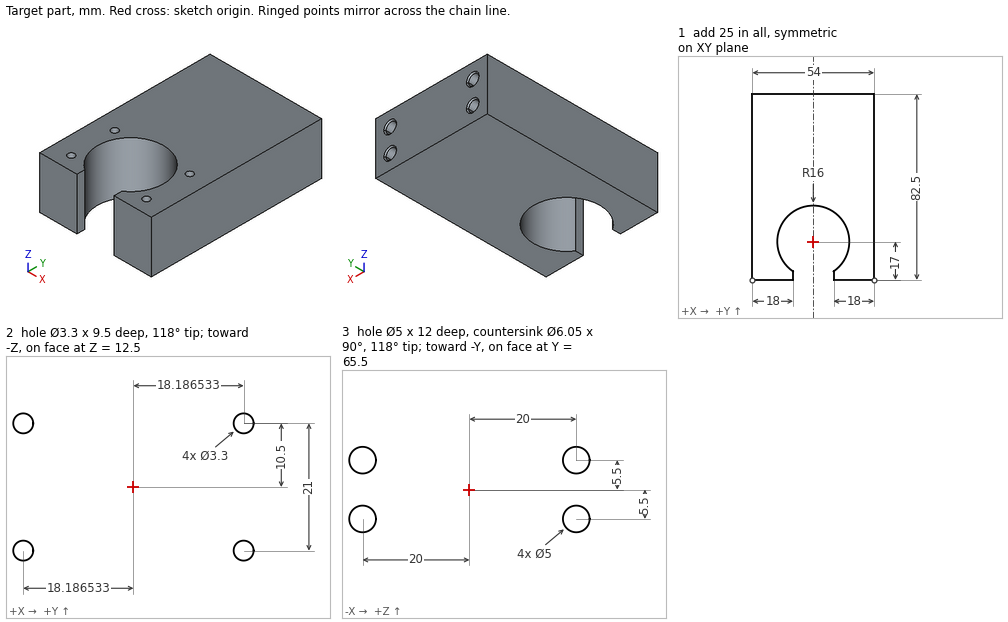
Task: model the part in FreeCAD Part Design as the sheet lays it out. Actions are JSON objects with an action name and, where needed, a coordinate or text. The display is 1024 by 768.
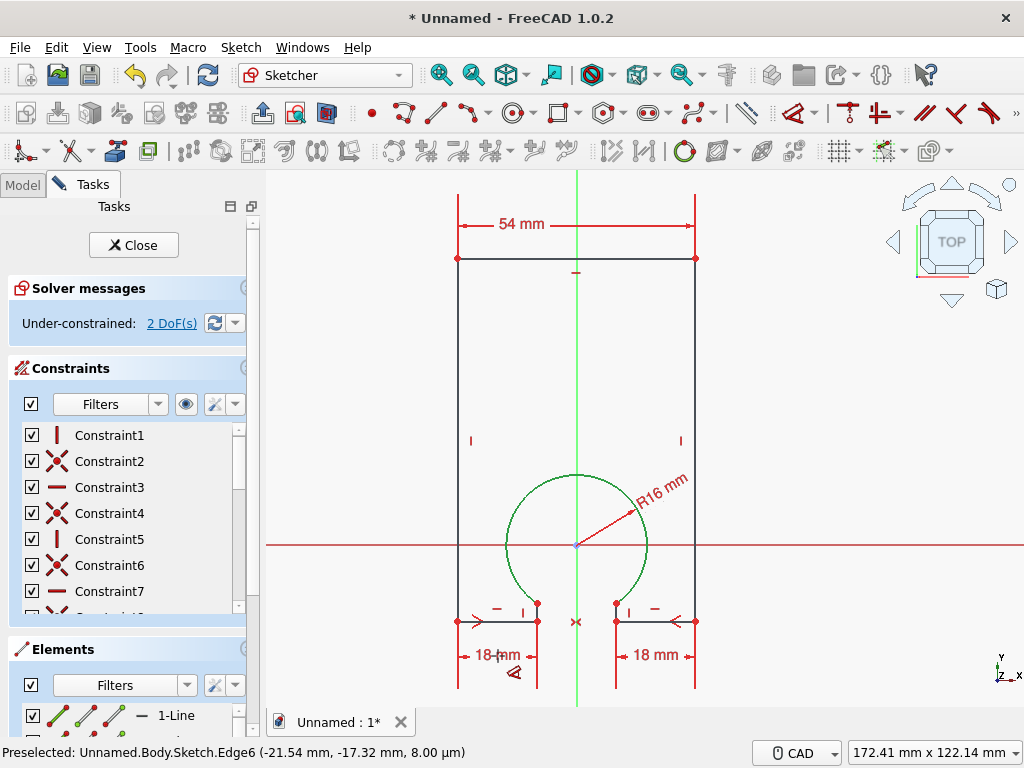
{"action": "left_click", "coordinate": [616, 622]}
{"action": "left_click", "coordinate": [650, 601]}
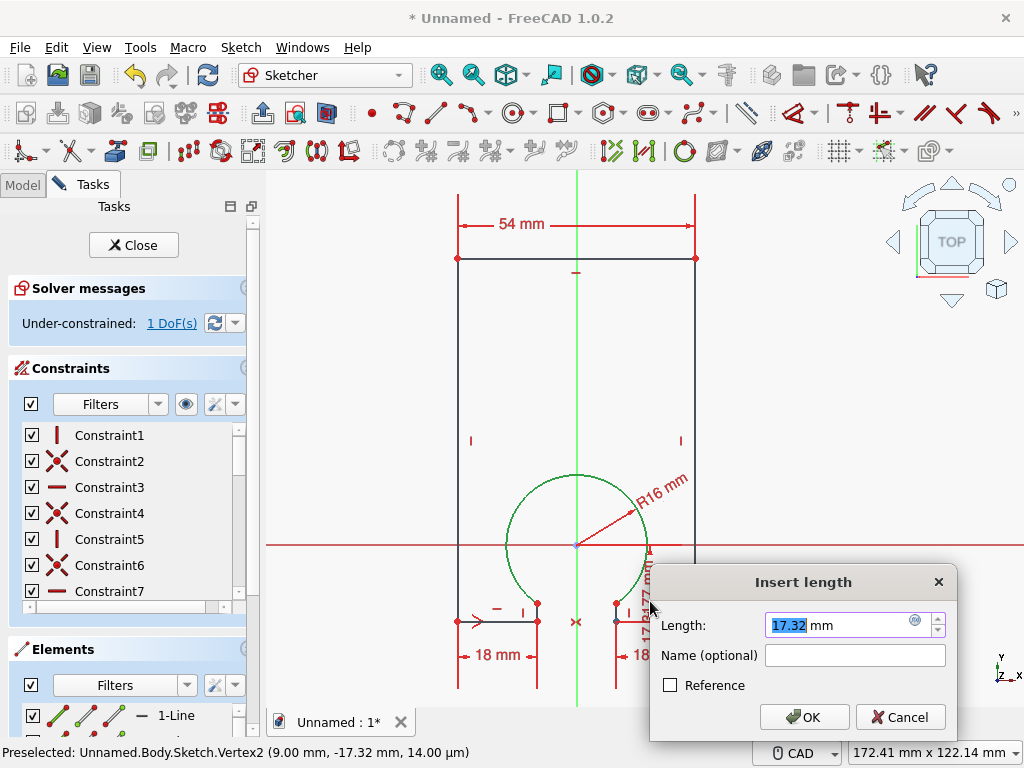
{"action": "type", "text": "17"}
{"action": "key", "text": "Return"}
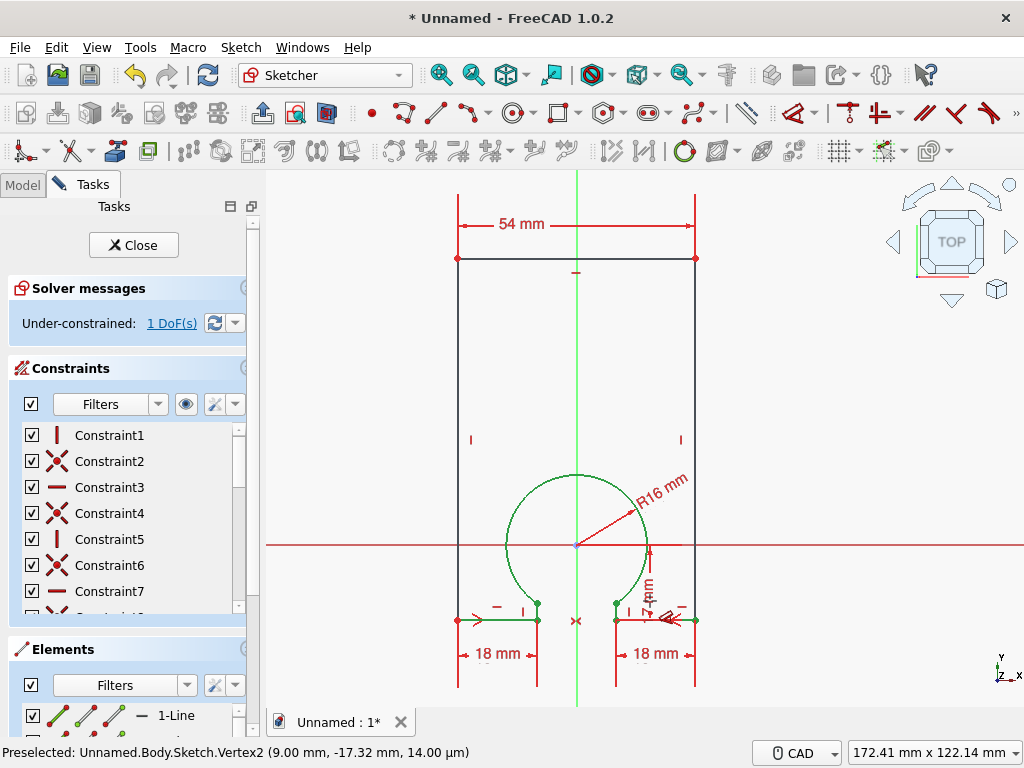
{"action": "left_click", "coordinate": [695, 512]}
{"action": "left_click", "coordinate": [729, 440]}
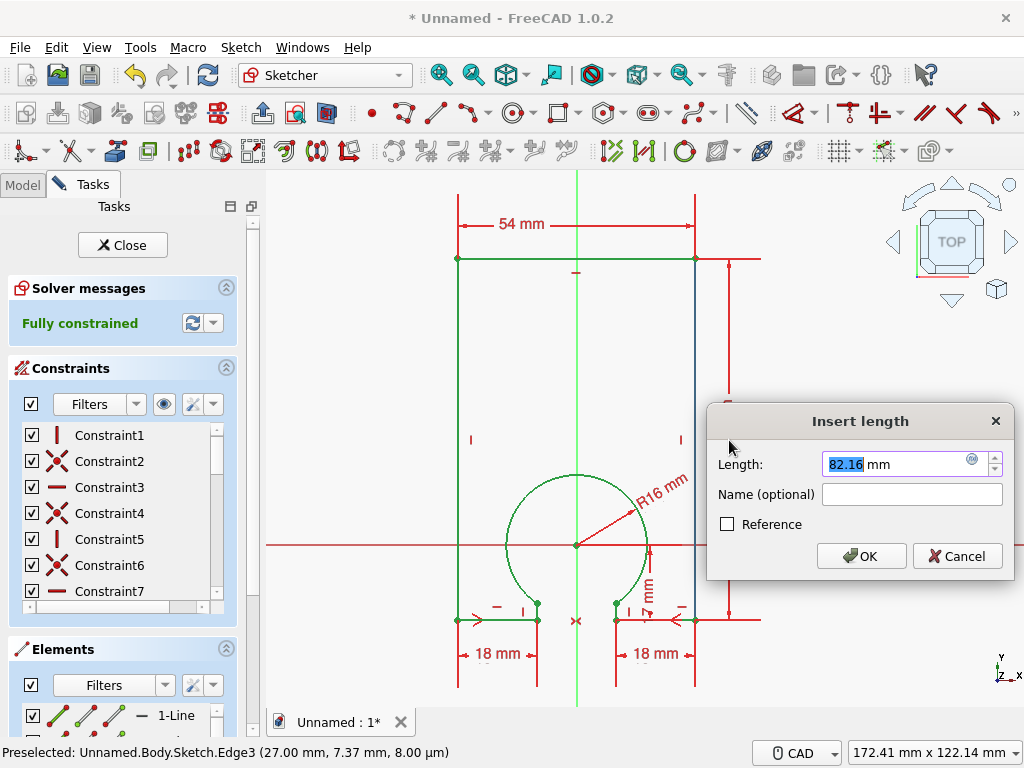
{"action": "type", "text": "82.5"}
{"action": "key", "text": "Return"}
{"action": "key", "text": "Escape"}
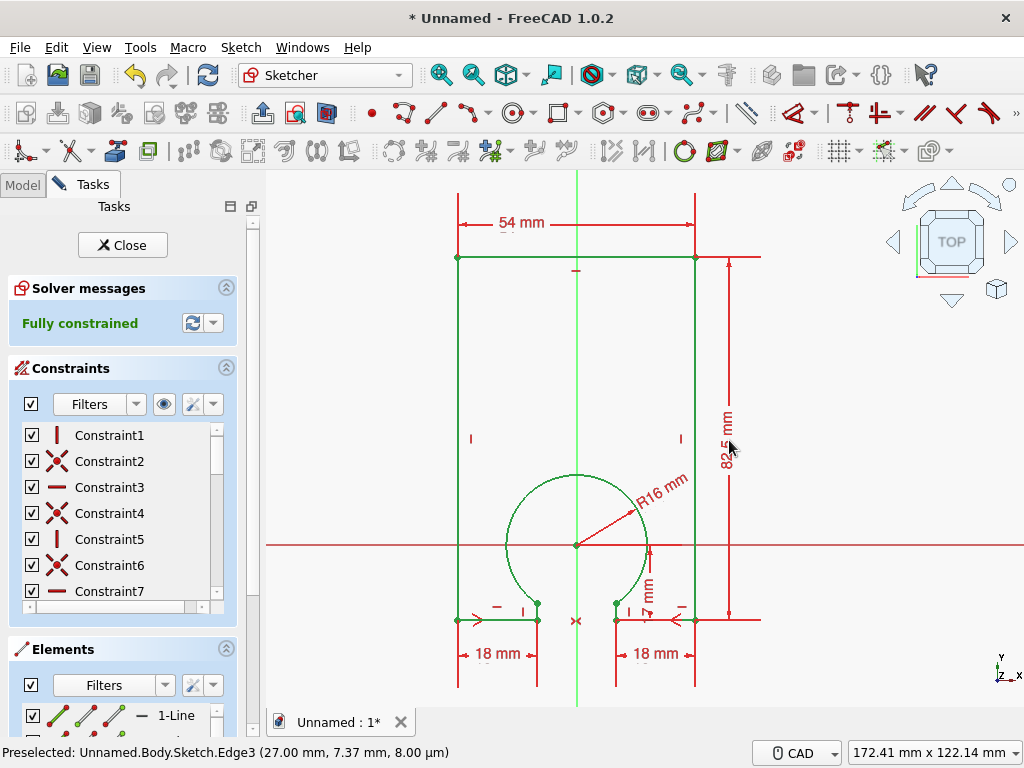
{"action": "left_click", "coordinate": [123, 245]}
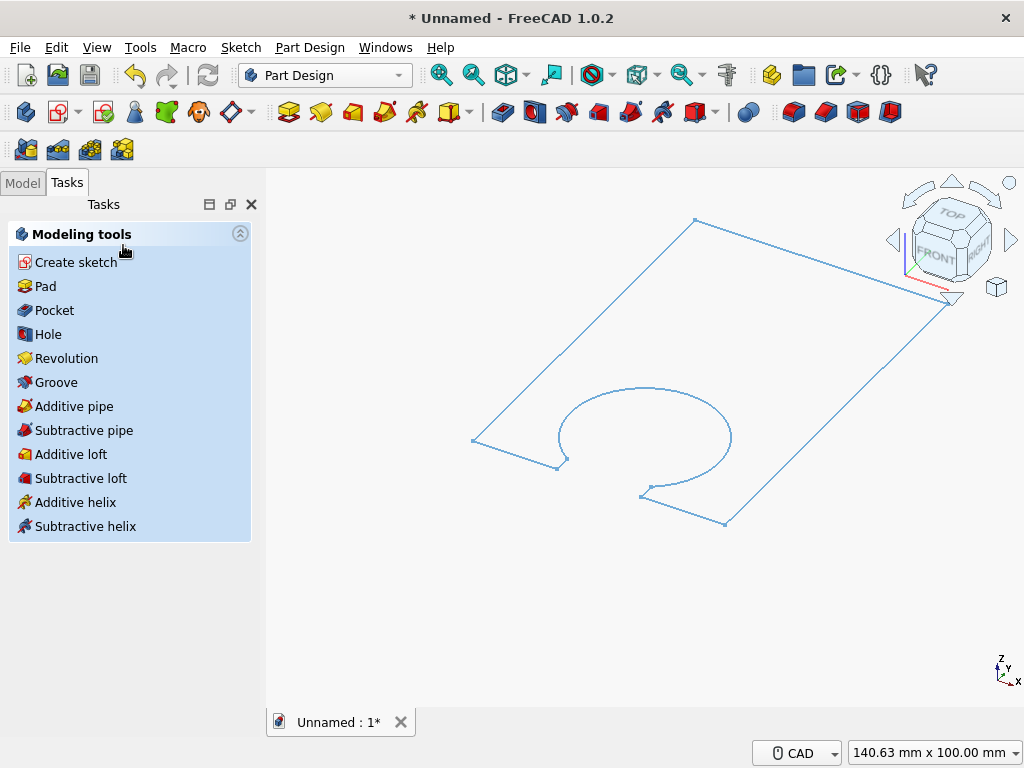
{"action": "left_click", "coordinate": [290, 112]}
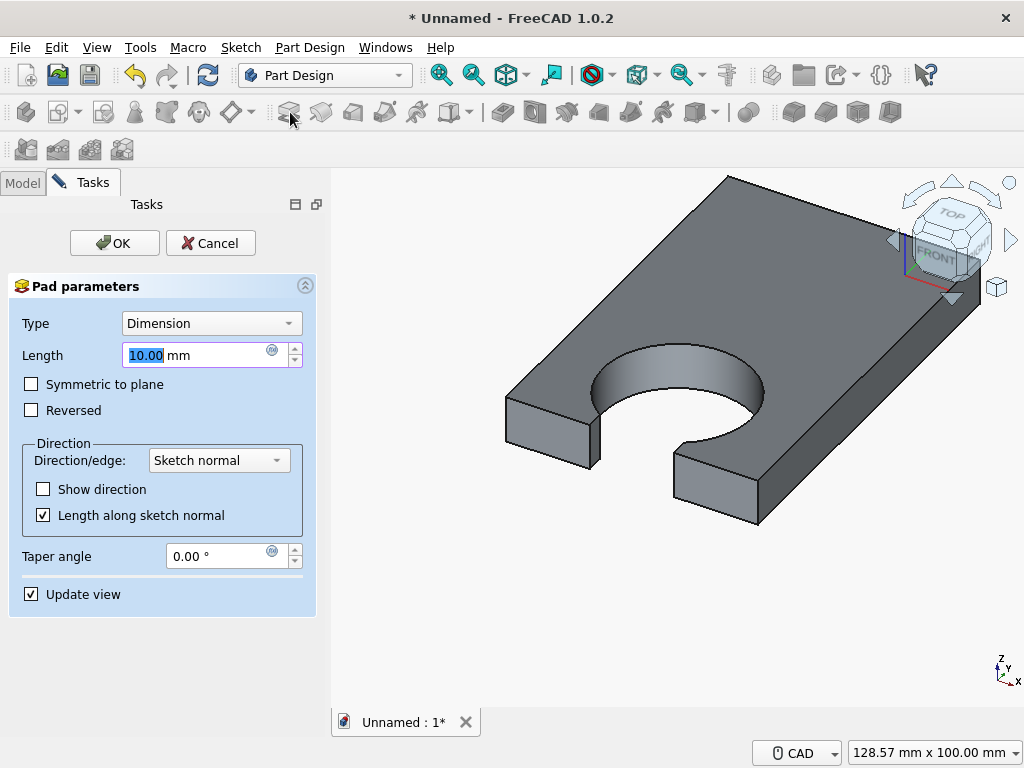
{"action": "type", "text": "25"}
{"action": "key", "text": "Tab"}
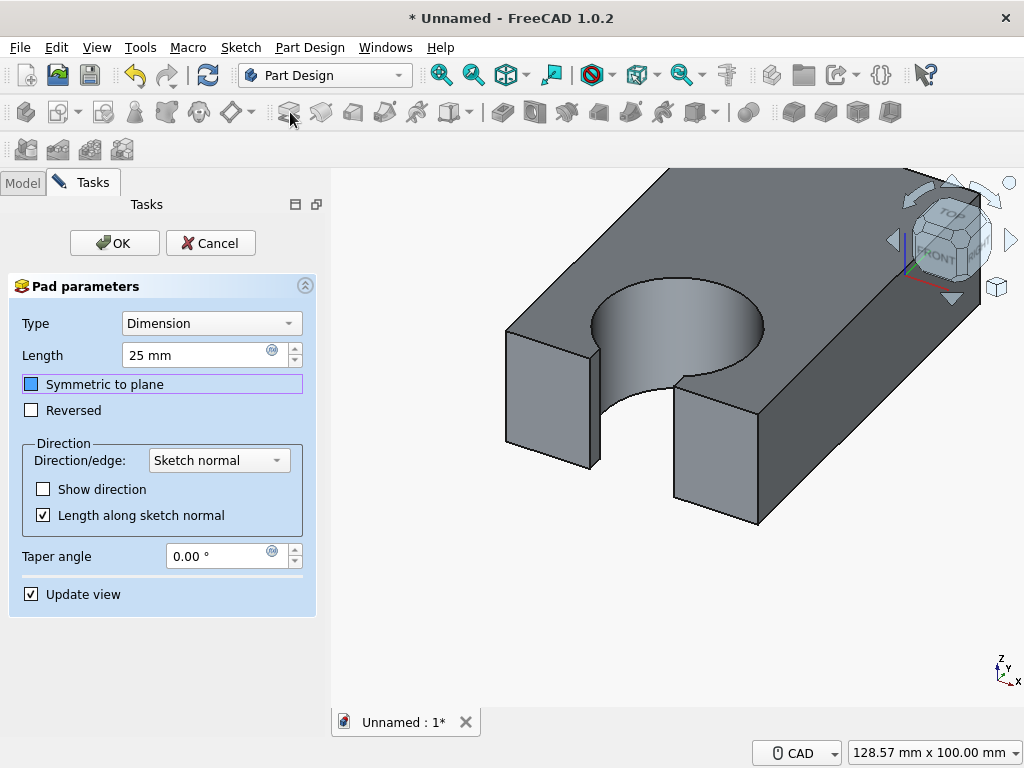
{"action": "left_click", "coordinate": [30, 384]}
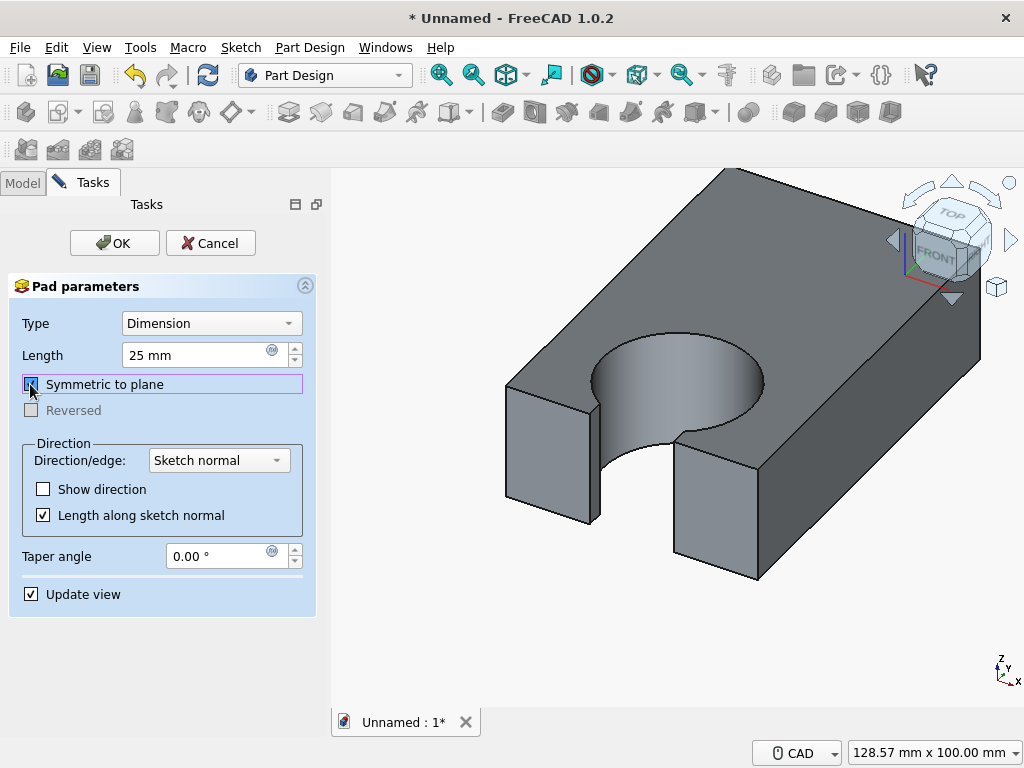
{"action": "left_click", "coordinate": [115, 243]}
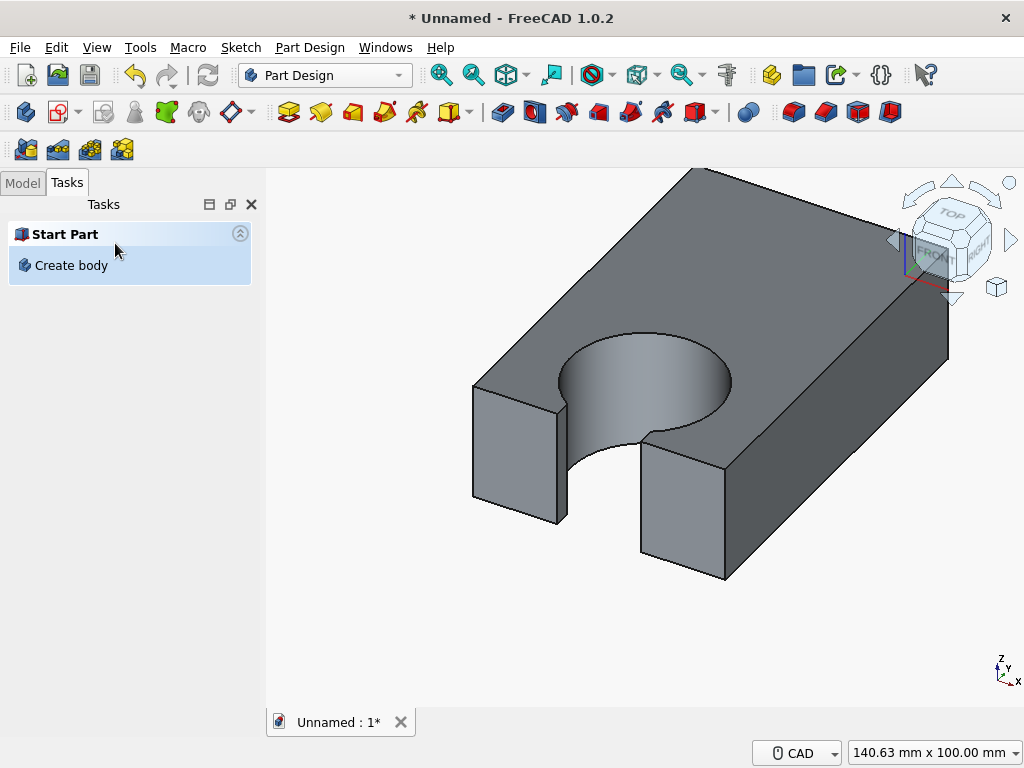
{"action": "left_click", "coordinate": [442, 76]}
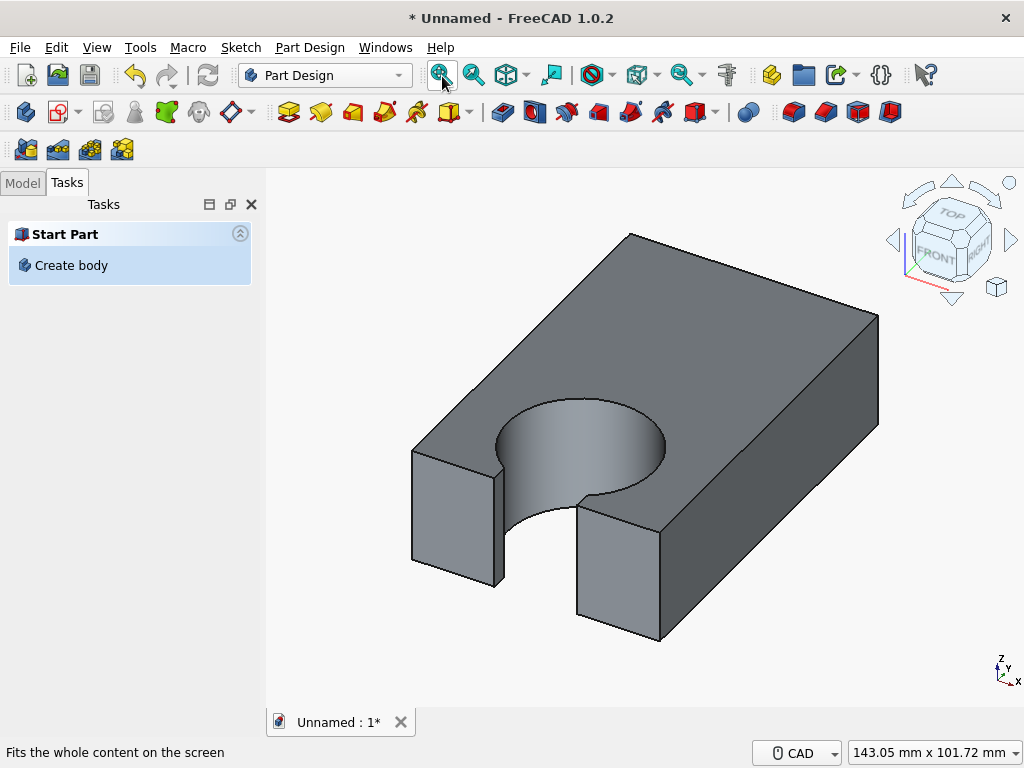
{"action": "left_click", "coordinate": [676, 351]}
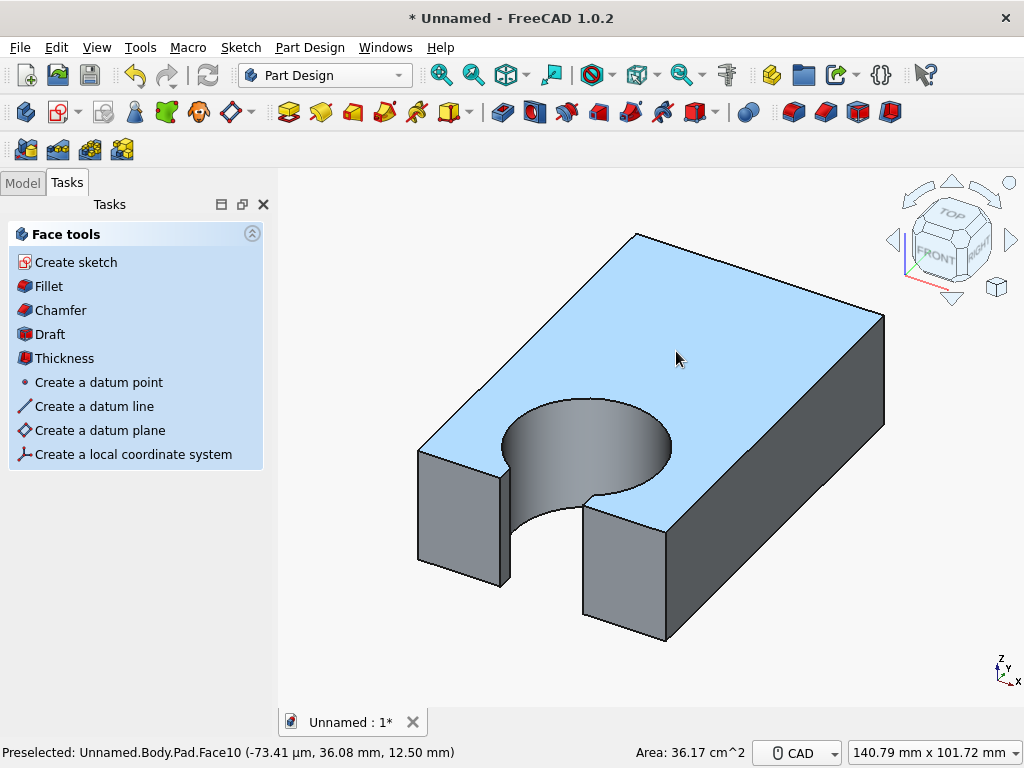
{"action": "left_click", "coordinate": [58, 112]}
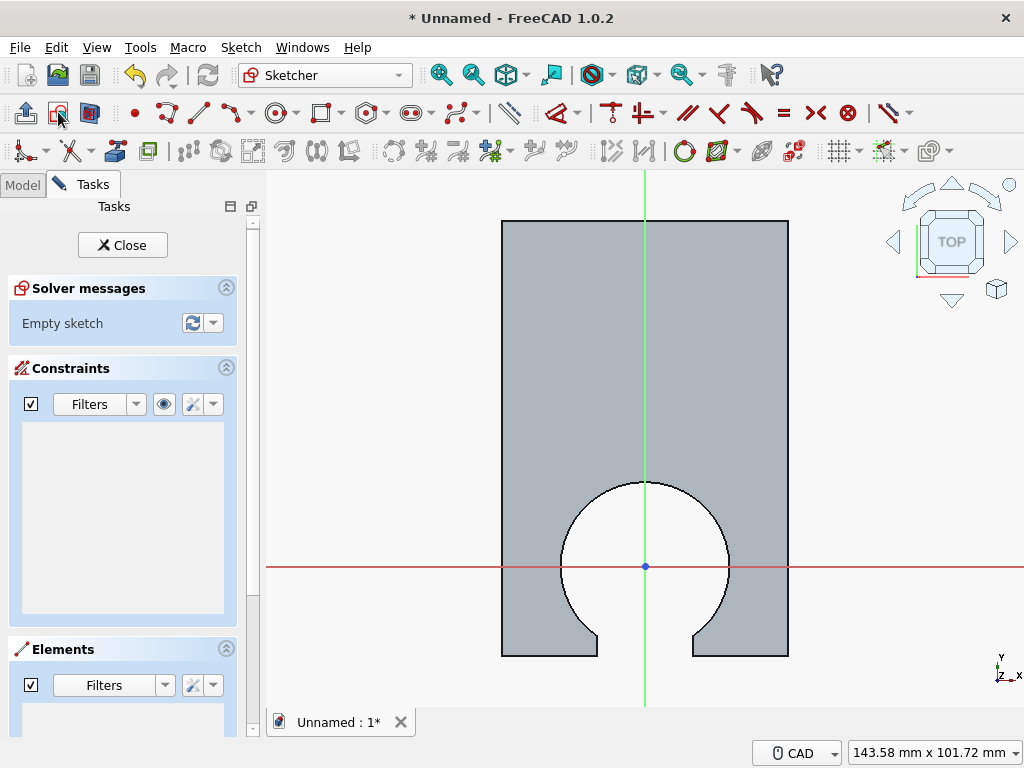
{"action": "scroll", "coordinate": [728, 679], "scroll_direction": "up", "scroll_amount": 3}